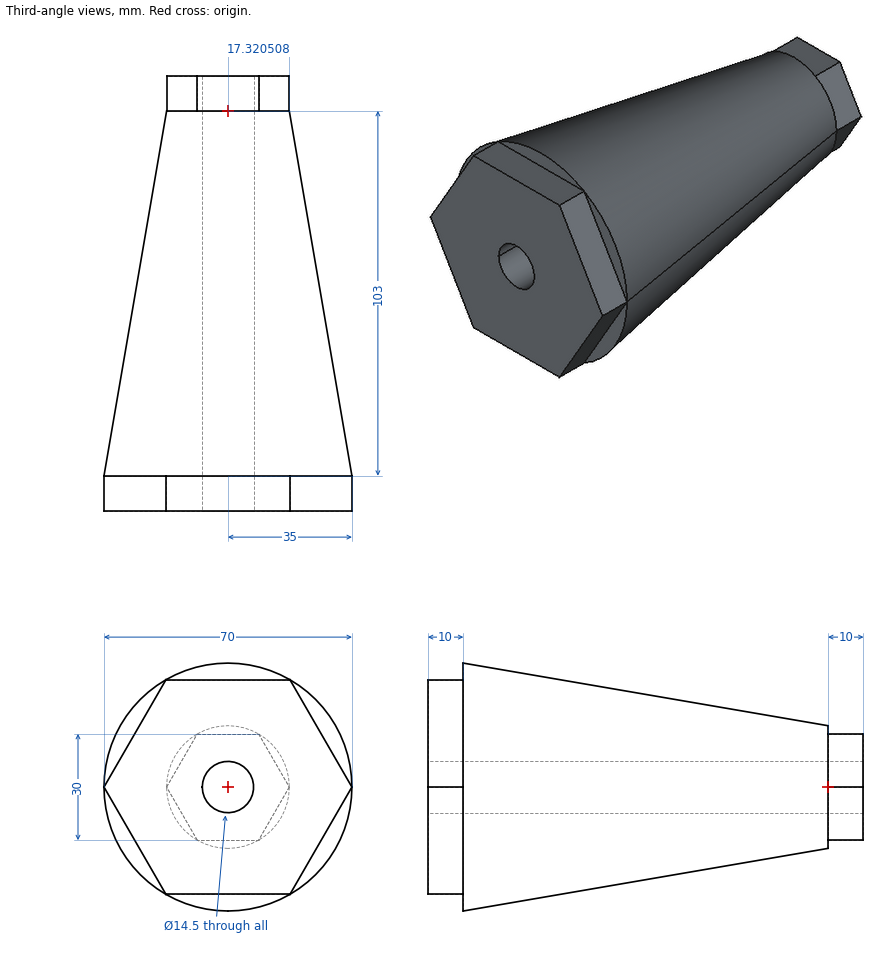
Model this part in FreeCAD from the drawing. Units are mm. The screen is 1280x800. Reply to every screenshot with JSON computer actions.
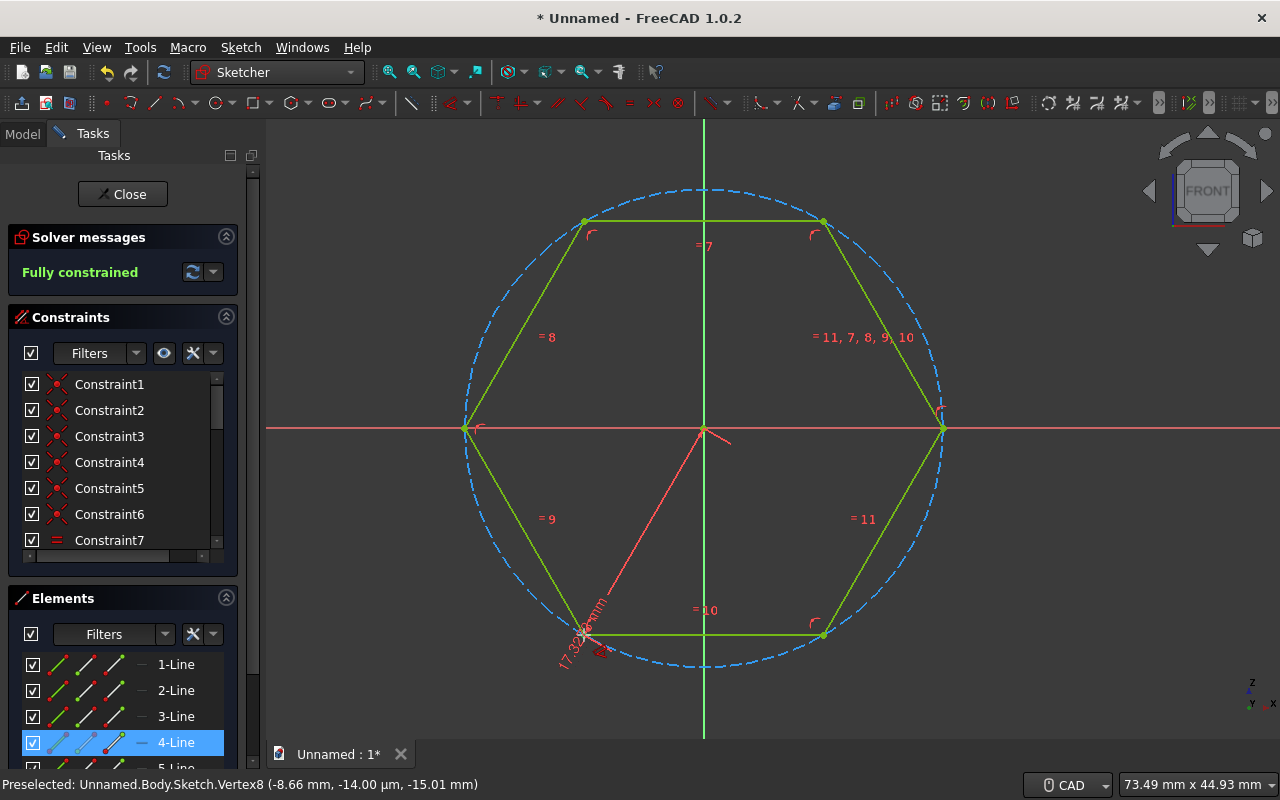
{"action": "left_click", "coordinate": [823, 221]}
{"action": "left_click", "coordinate": [857, 333]}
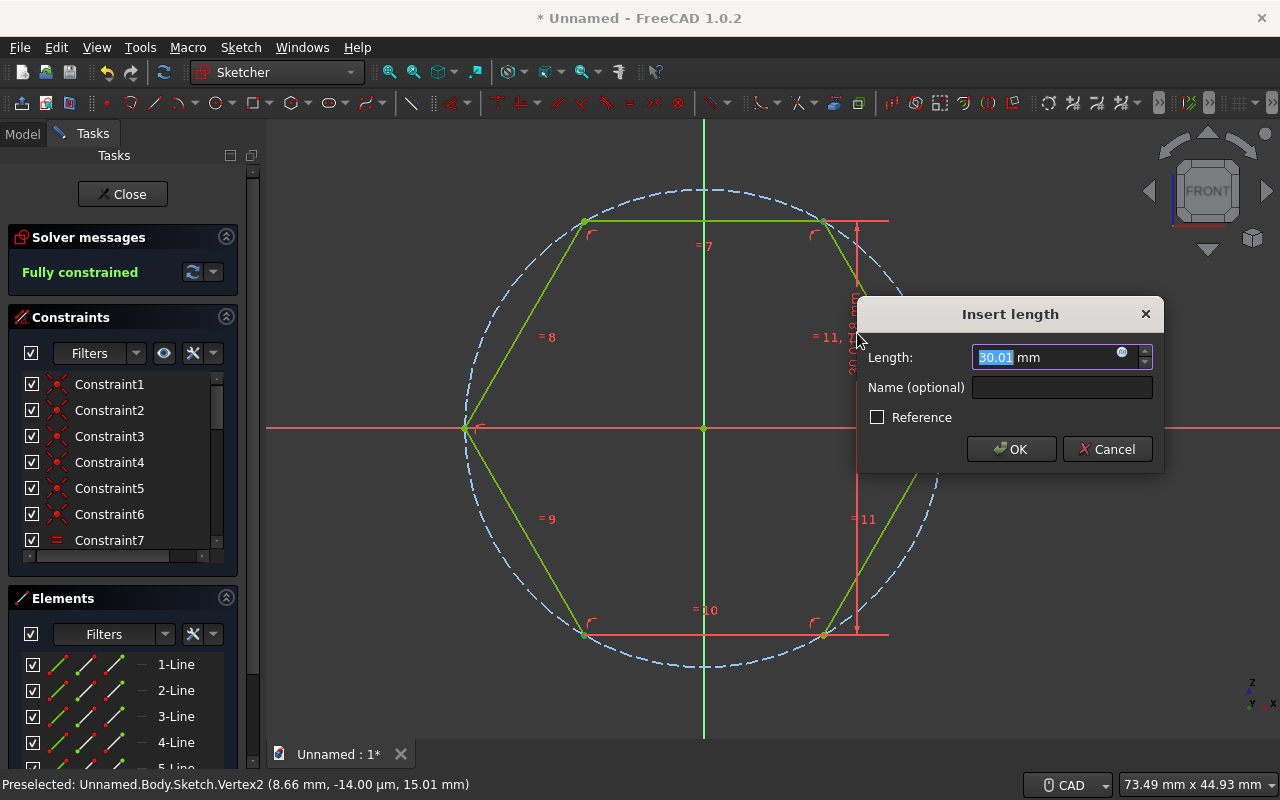
{"action": "type", "text": "30"}
{"action": "key", "text": "Return"}
{"action": "key", "text": "Escape"}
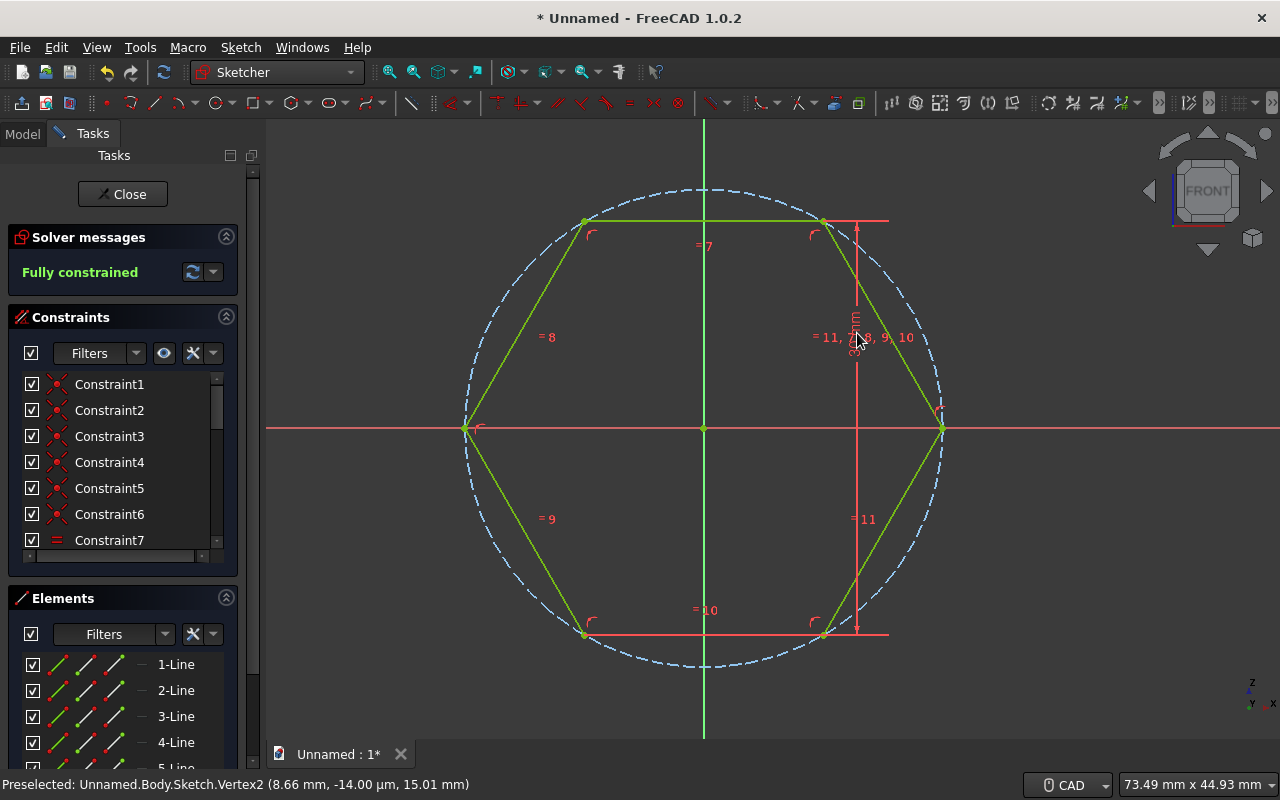
{"action": "left_click", "coordinate": [123, 194]}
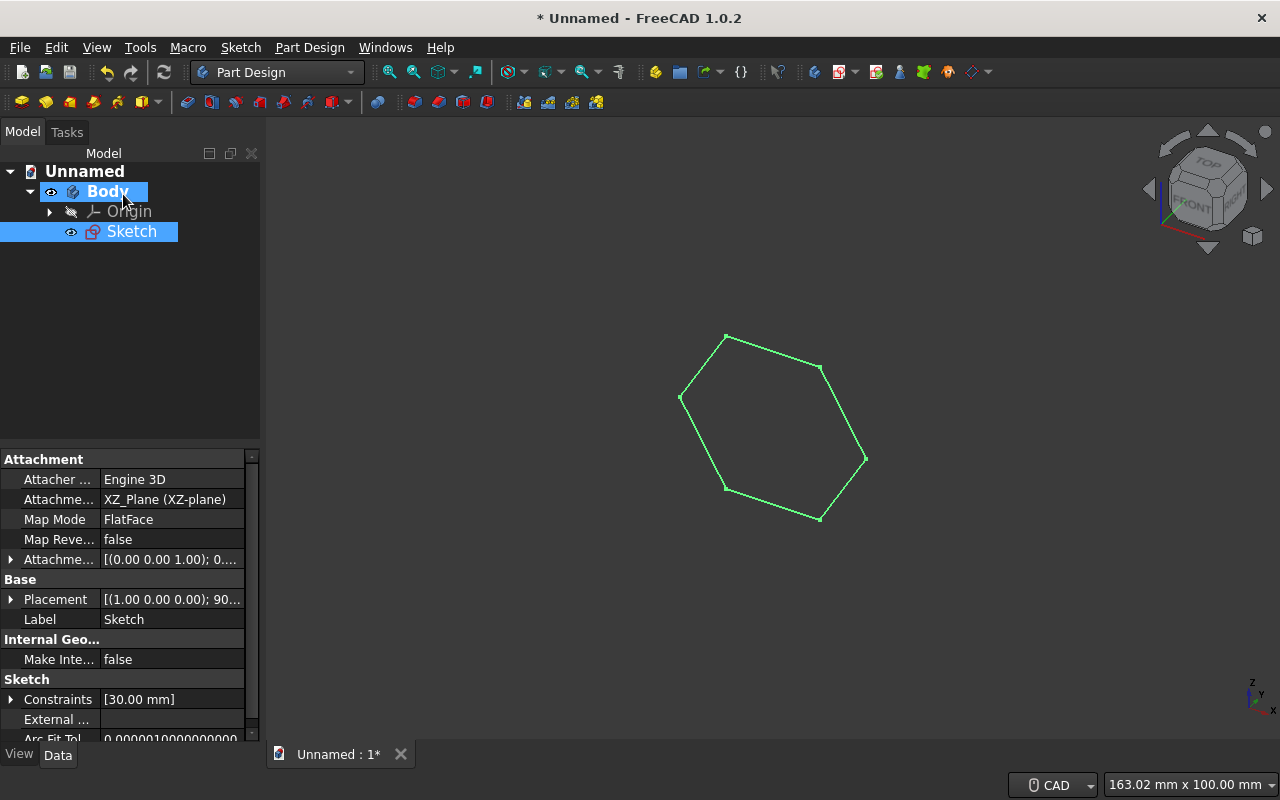
{"action": "left_click", "coordinate": [22, 102]}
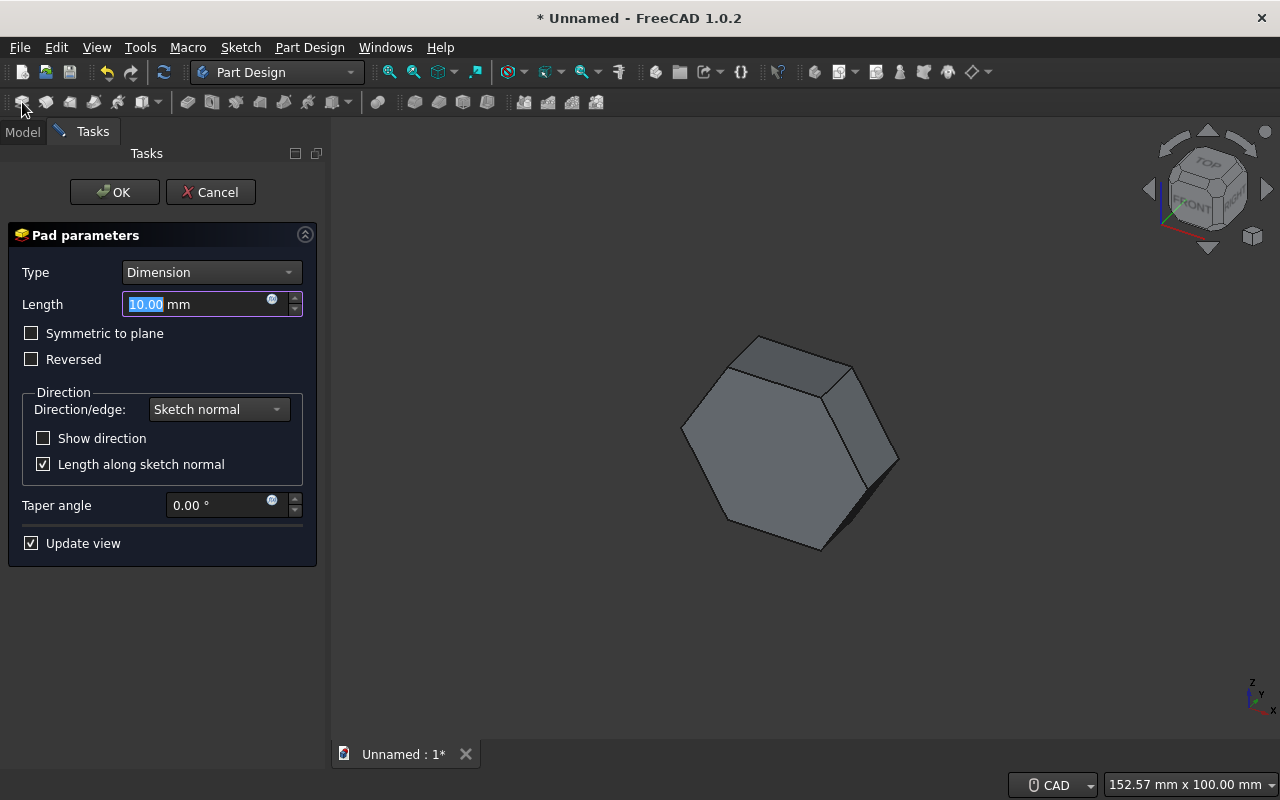
{"action": "type", "text": "10"}
{"action": "key", "text": "Tab"}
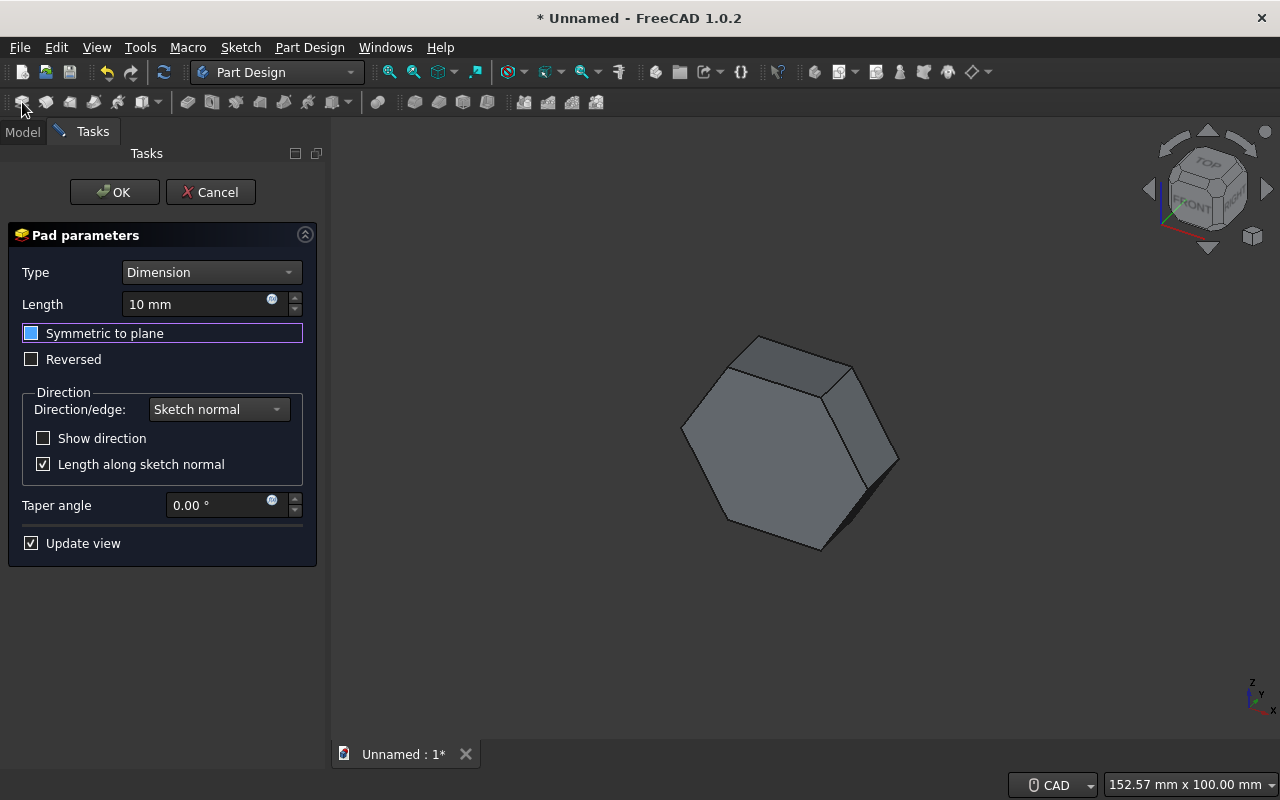
{"action": "left_click", "coordinate": [30, 359]}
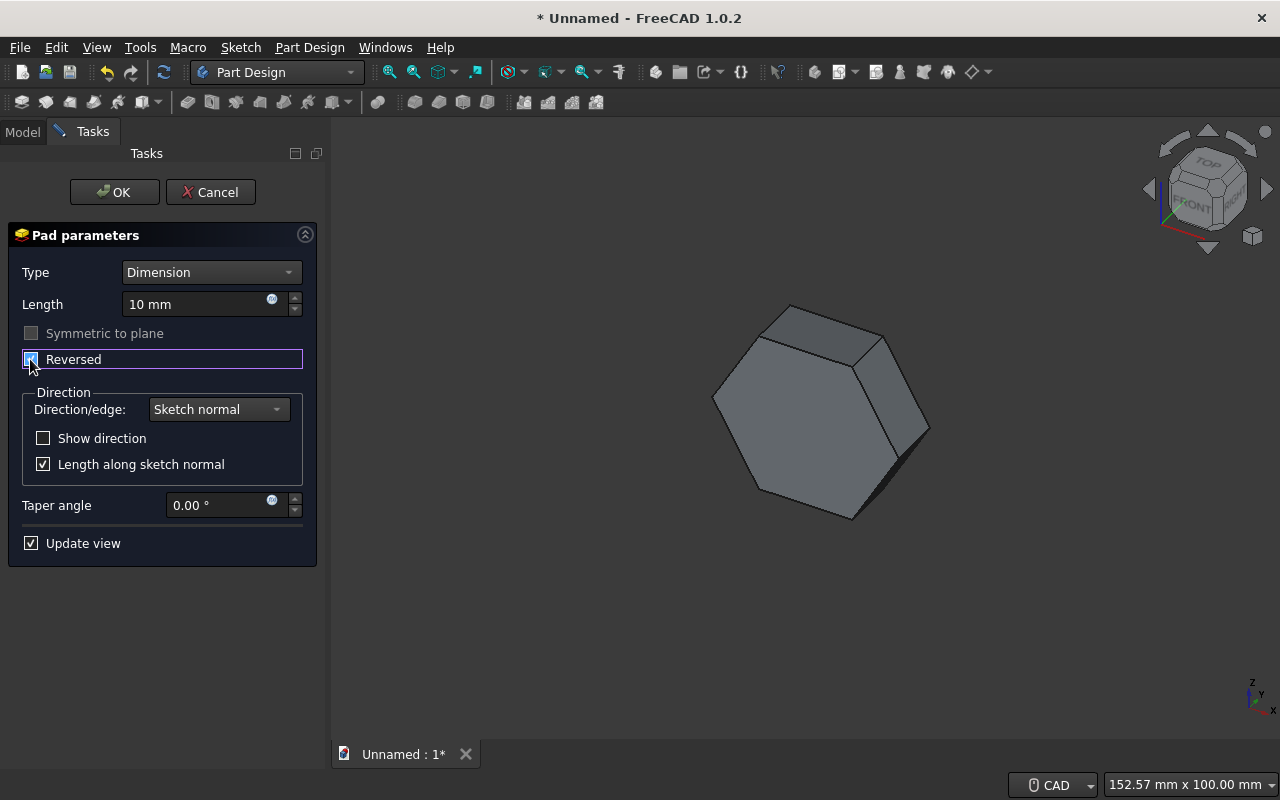
{"action": "left_click", "coordinate": [115, 192]}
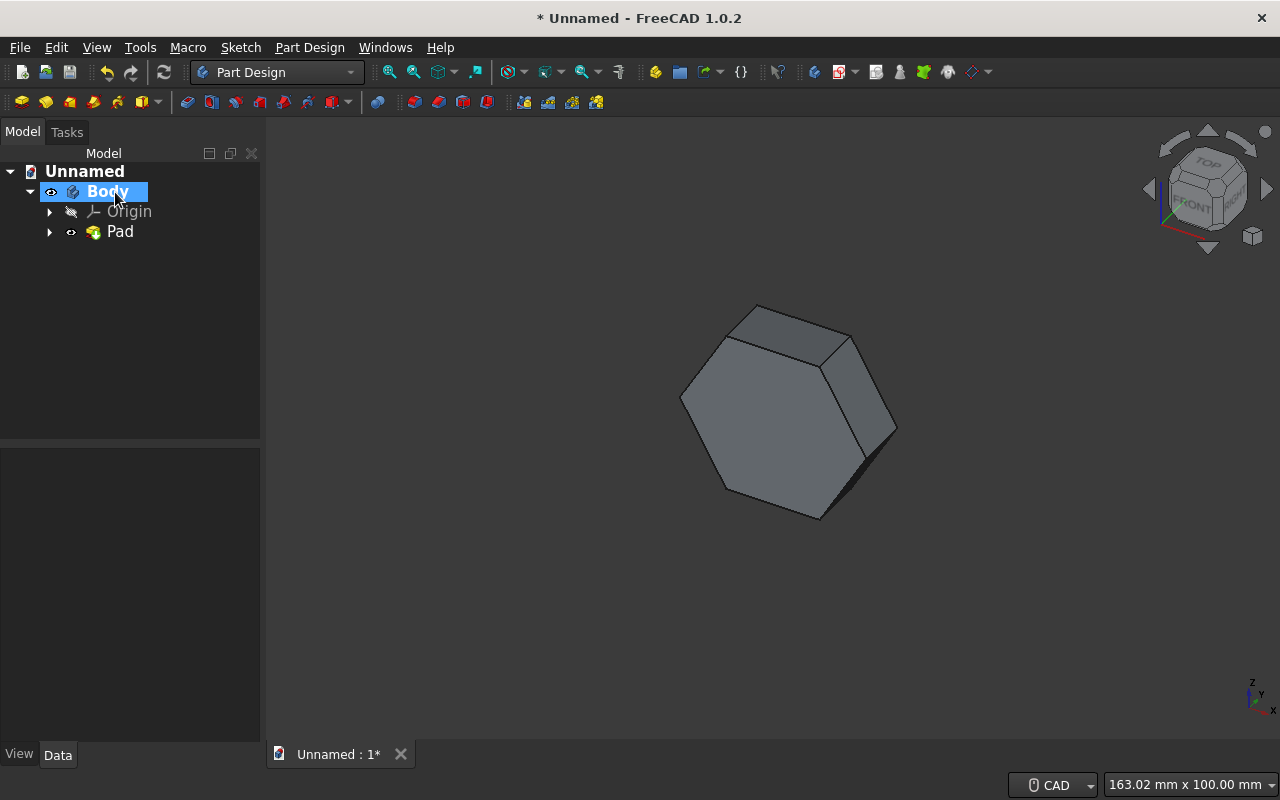
{"action": "left_click", "coordinate": [390, 72]}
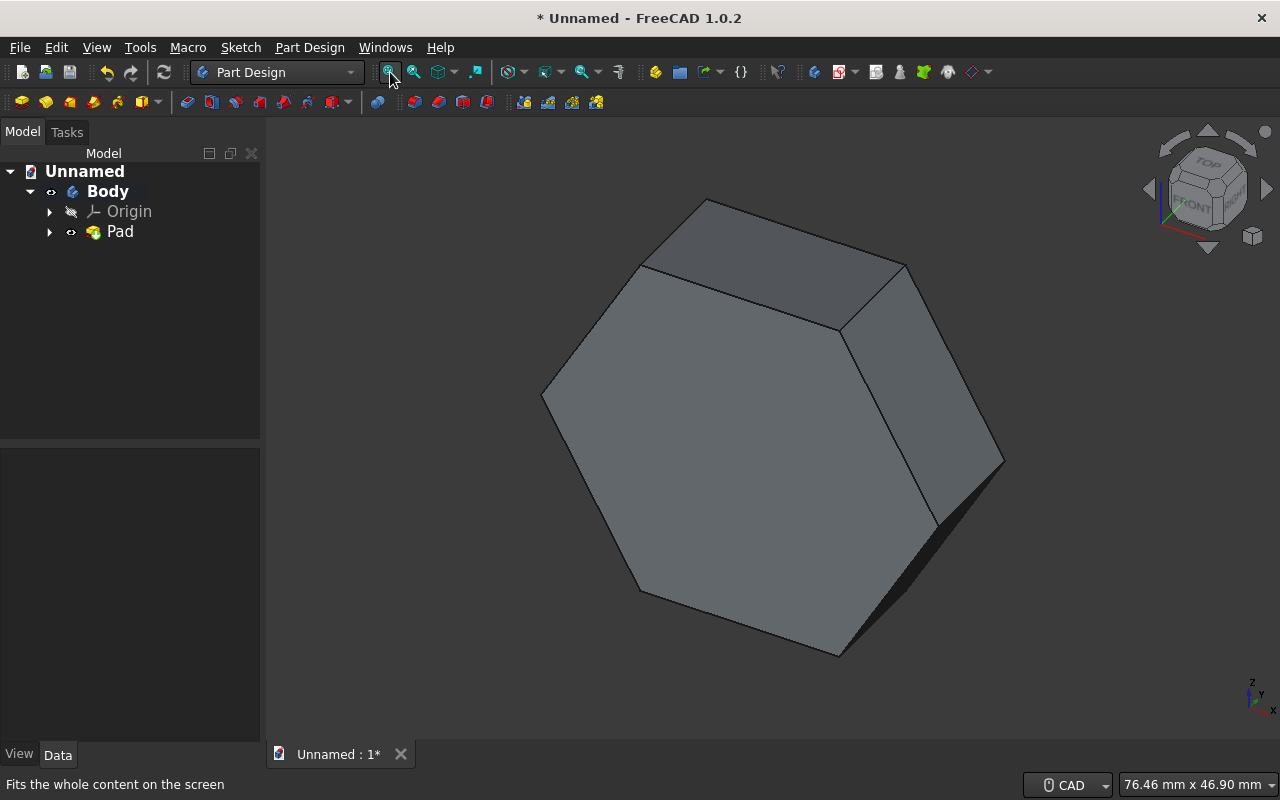
{"action": "left_click", "coordinate": [840, 72]}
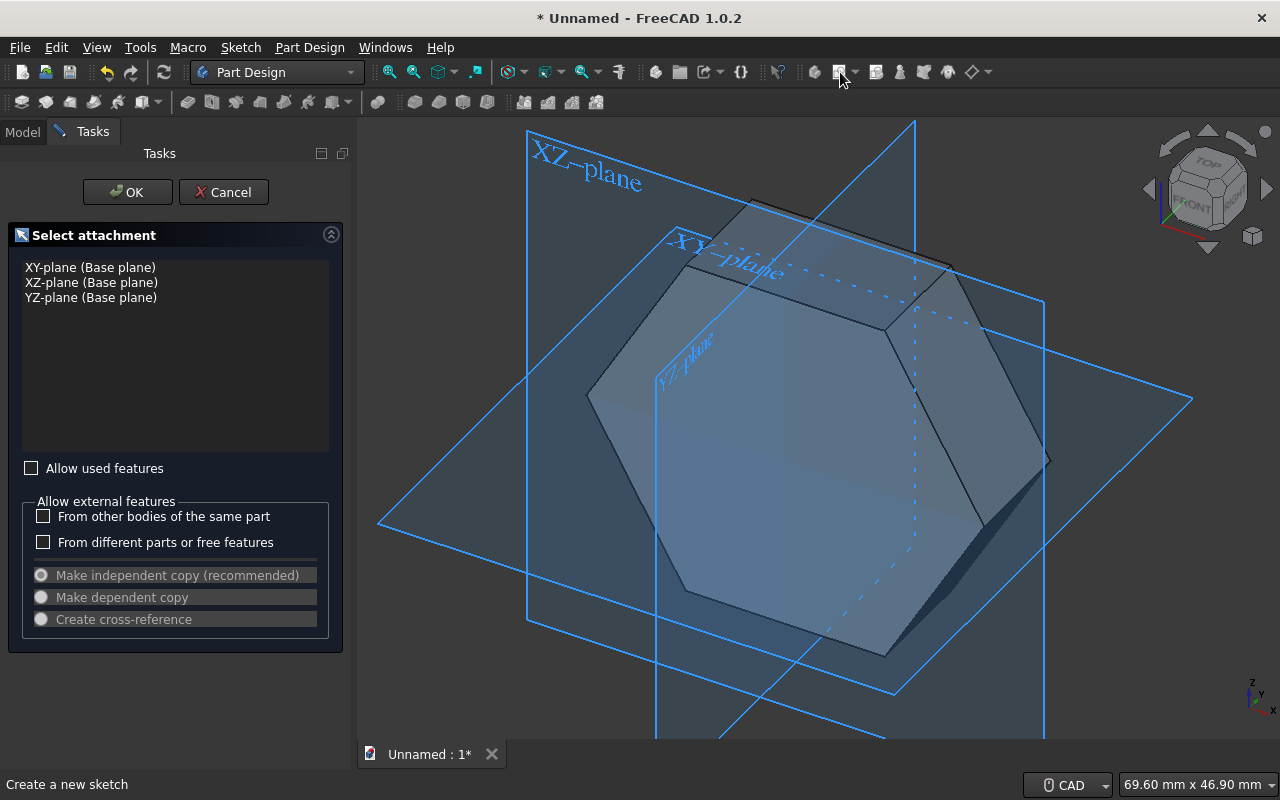
{"action": "left_click", "coordinate": [82, 268]}